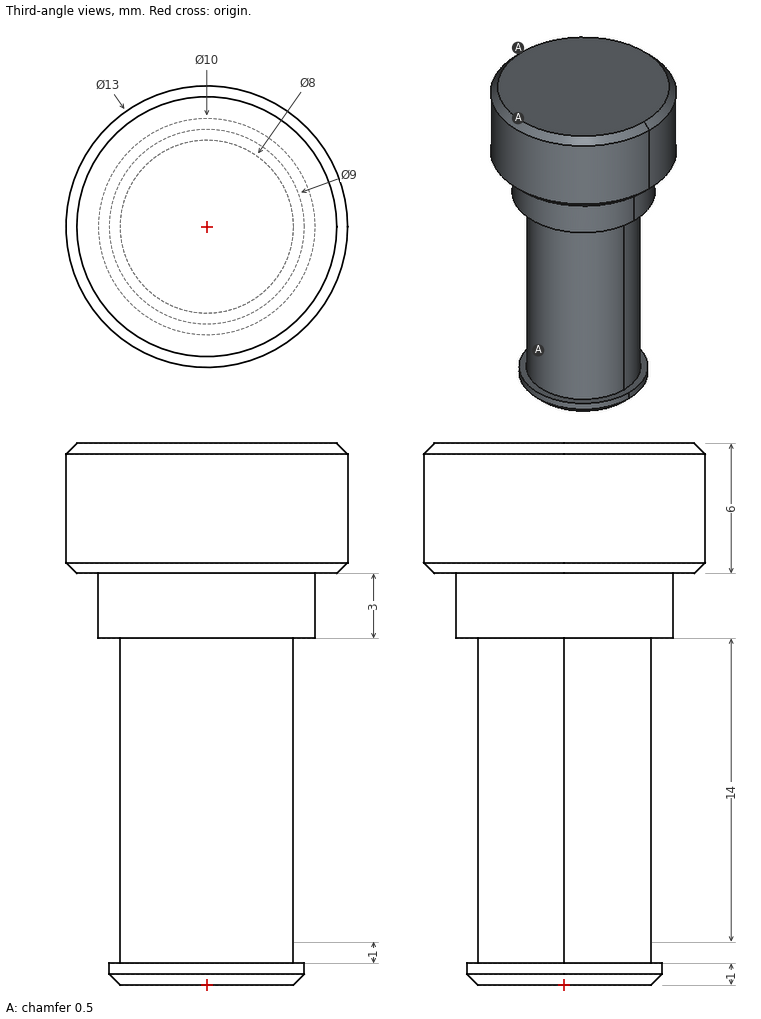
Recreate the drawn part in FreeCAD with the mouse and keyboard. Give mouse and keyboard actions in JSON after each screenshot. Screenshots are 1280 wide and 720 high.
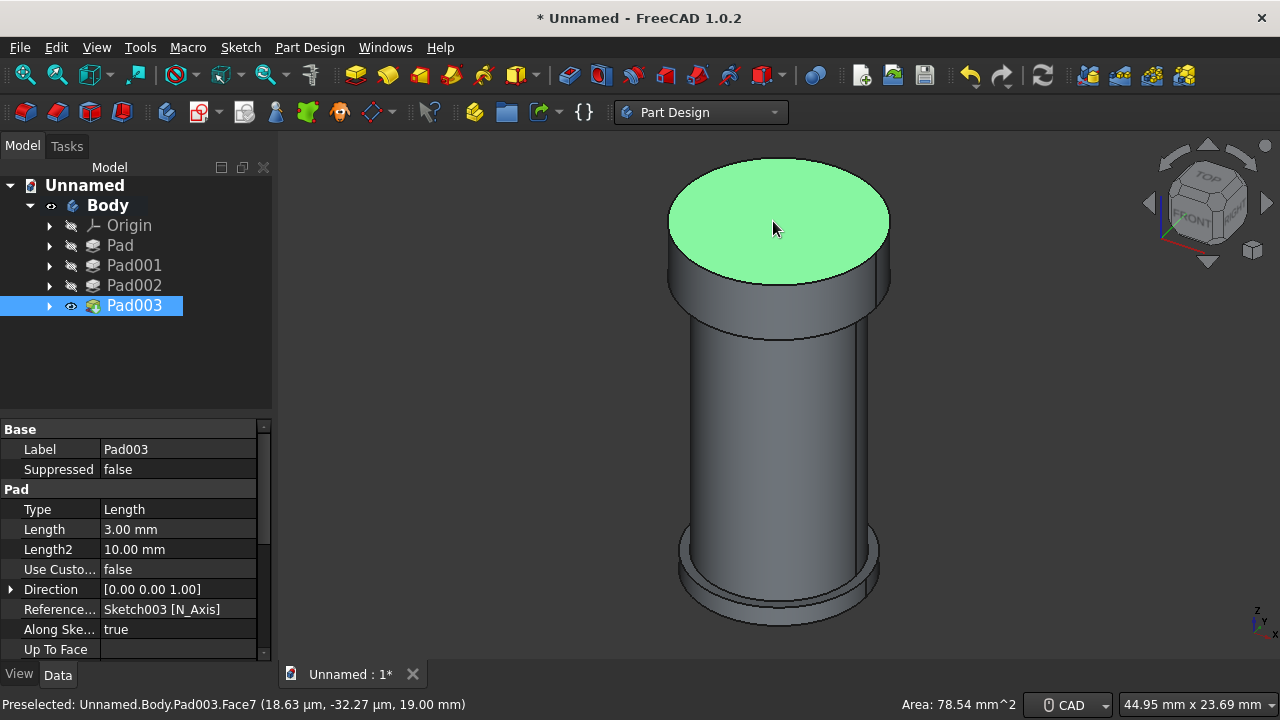
{"action": "left_click", "coordinate": [200, 112]}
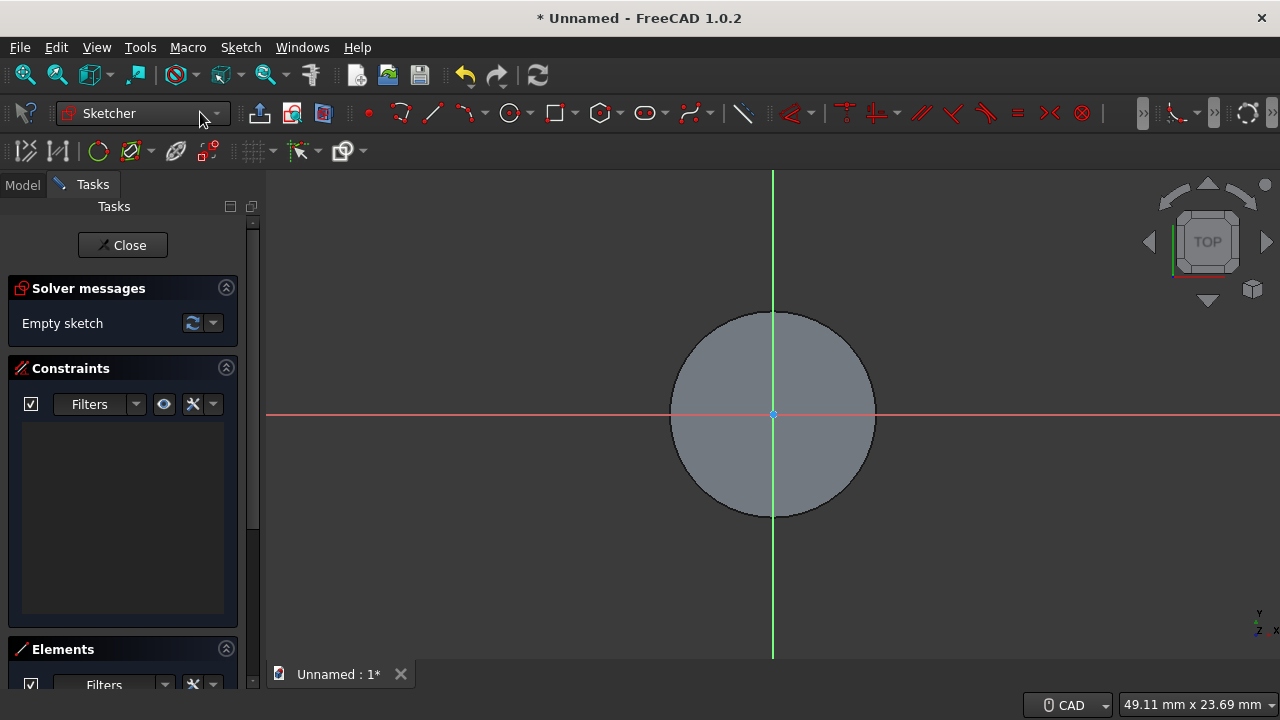
{"action": "left_click", "coordinate": [510, 114]}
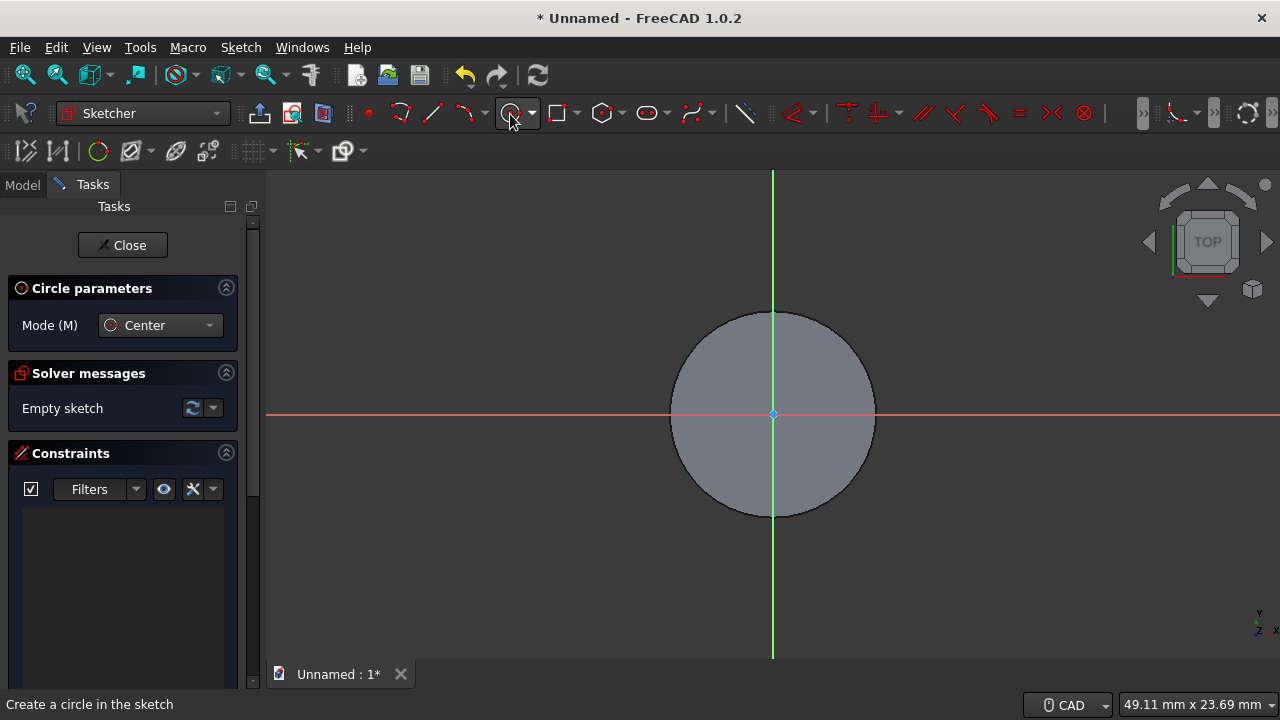
{"action": "left_click", "coordinate": [773, 414]}
{"action": "mouse_move", "coordinate": [868, 320]}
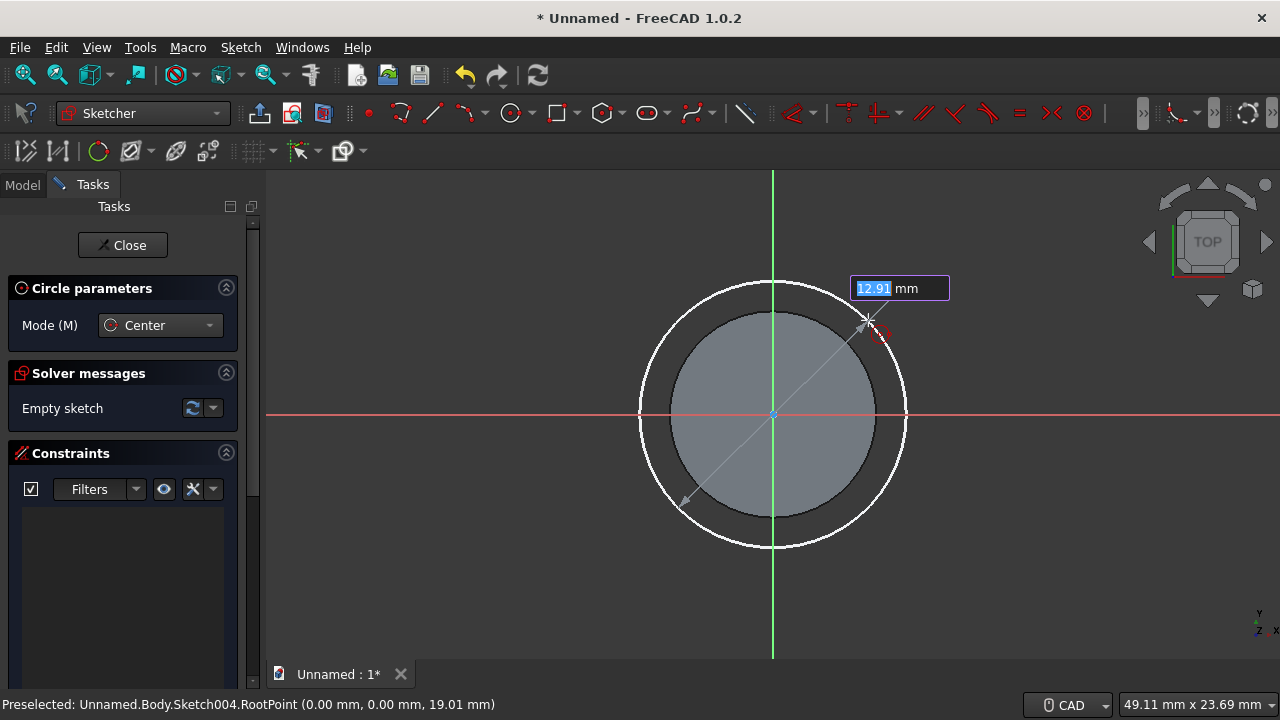
{"action": "type", "text": "13"}
{"action": "key", "text": "Return"}
{"action": "key", "text": "Escape"}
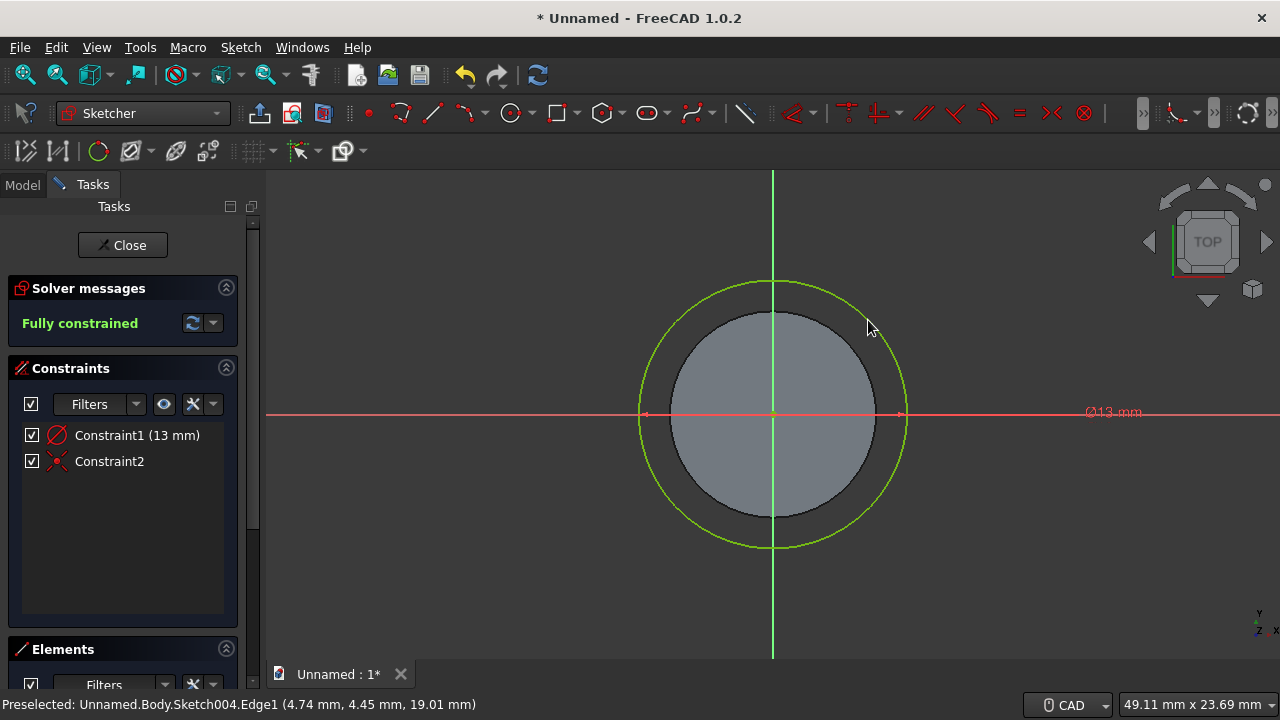
{"action": "left_click", "coordinate": [123, 245]}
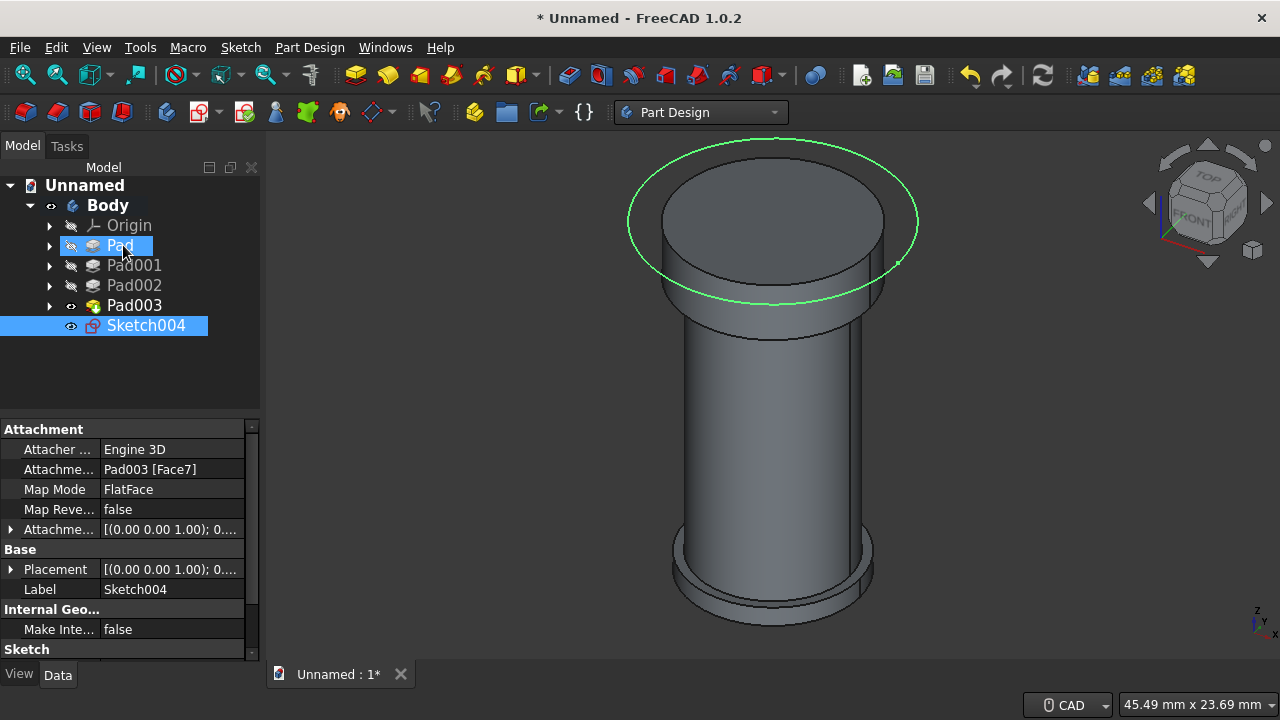
{"action": "left_click", "coordinate": [356, 76]}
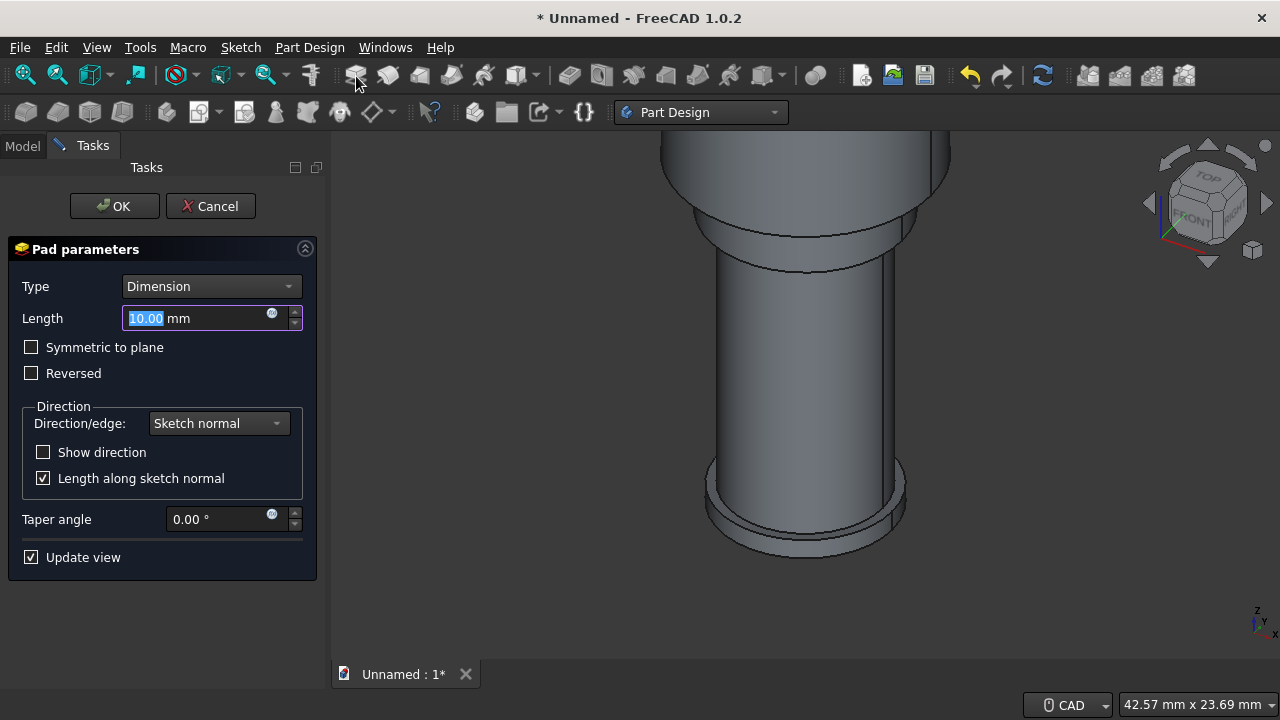
{"action": "type", "text": "6"}
{"action": "key", "text": "Tab"}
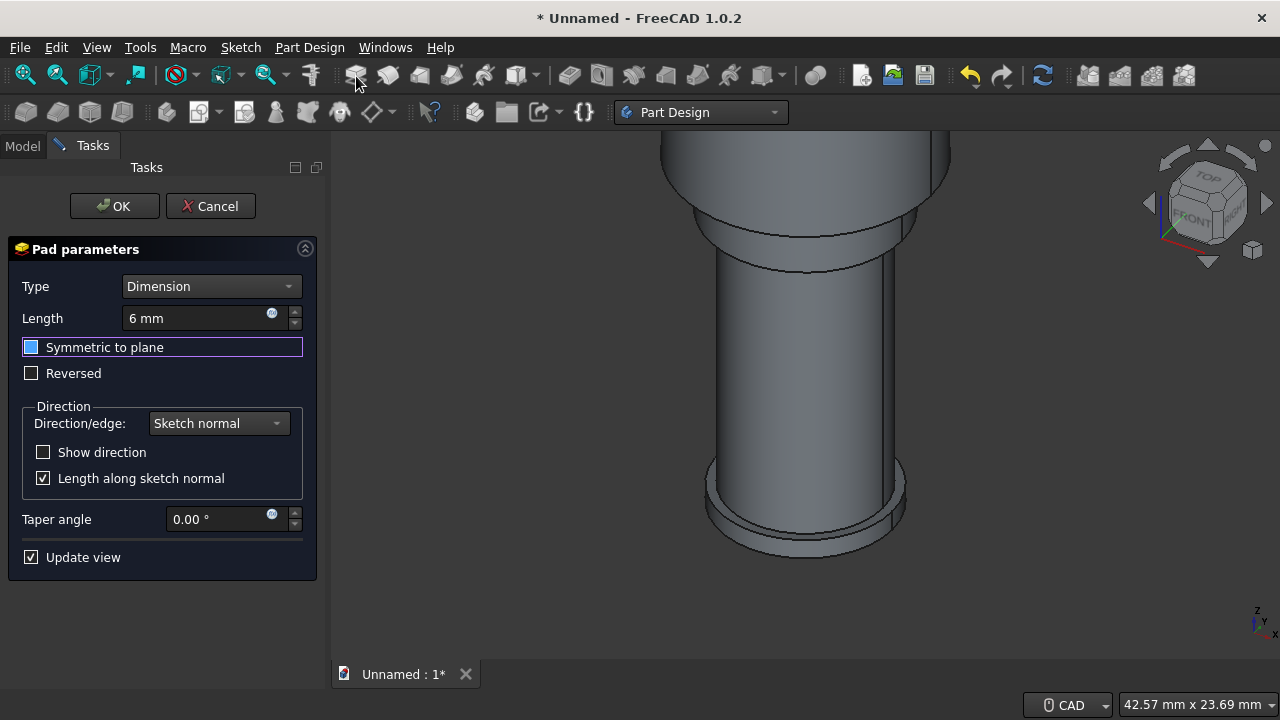
{"action": "left_click", "coordinate": [115, 206]}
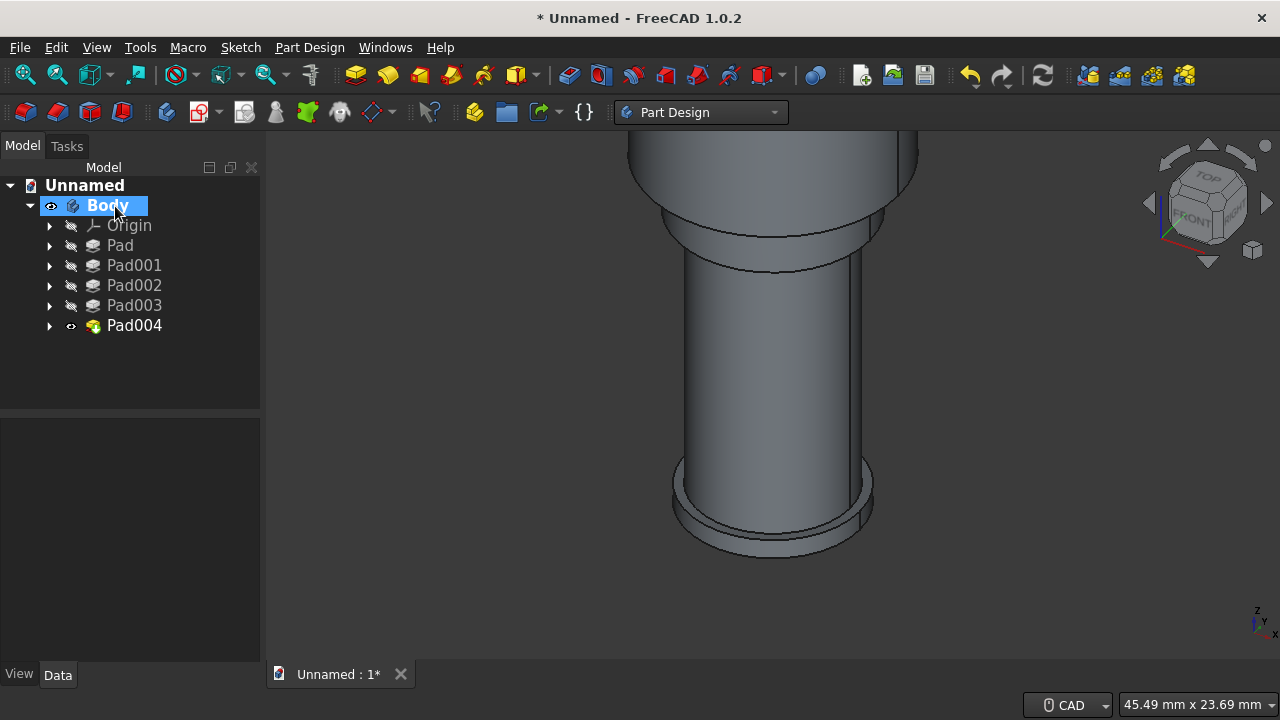
{"action": "left_click", "coordinate": [26, 76]}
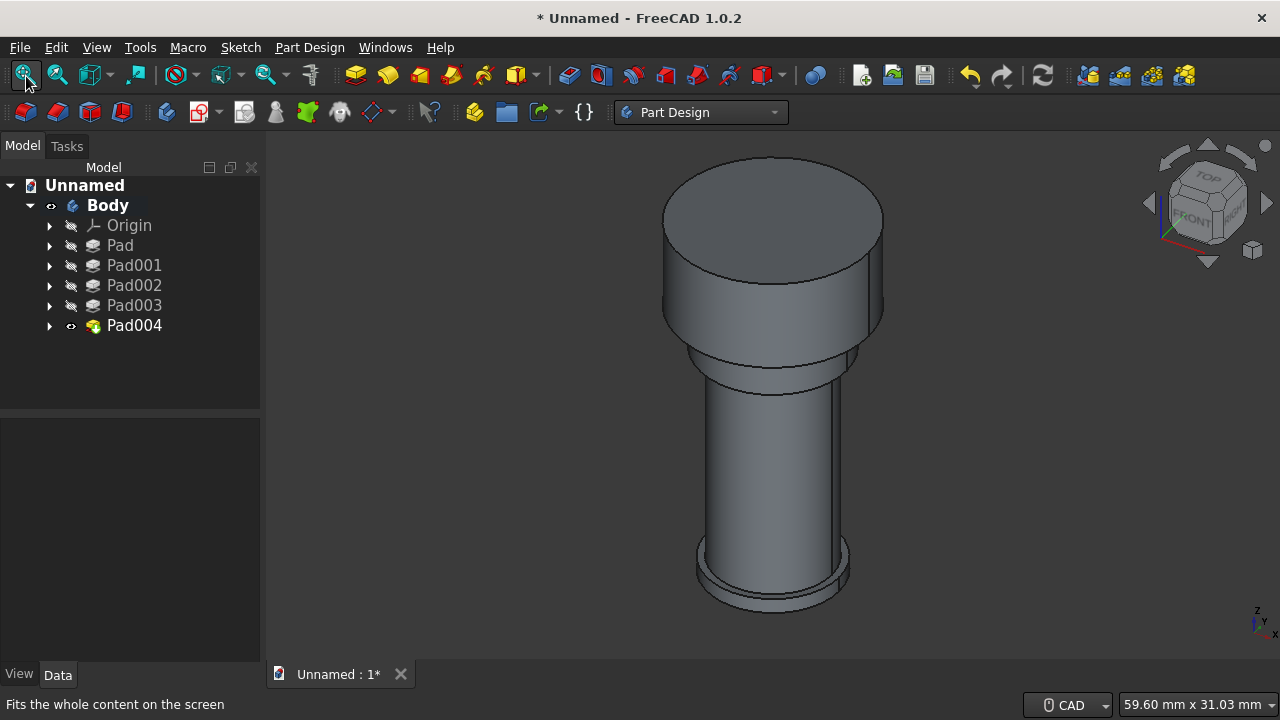
{"action": "left_click", "coordinate": [663, 226]}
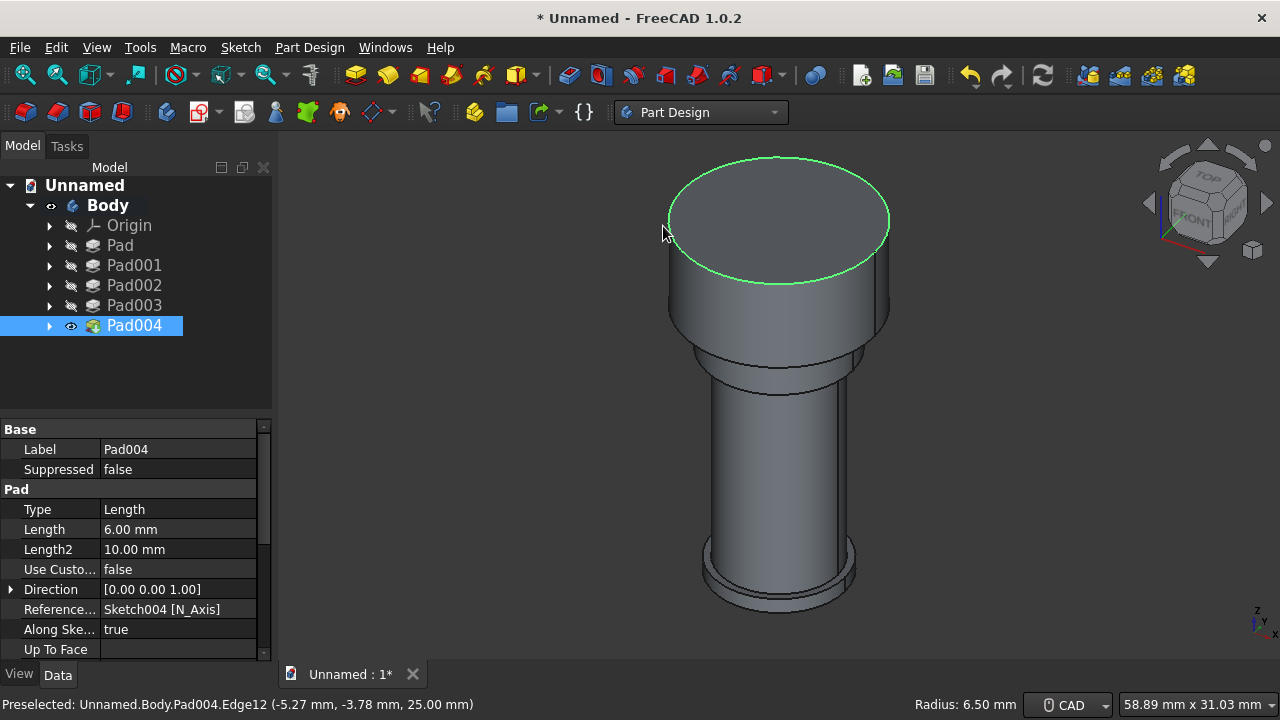
{"action": "key", "text": "0"}